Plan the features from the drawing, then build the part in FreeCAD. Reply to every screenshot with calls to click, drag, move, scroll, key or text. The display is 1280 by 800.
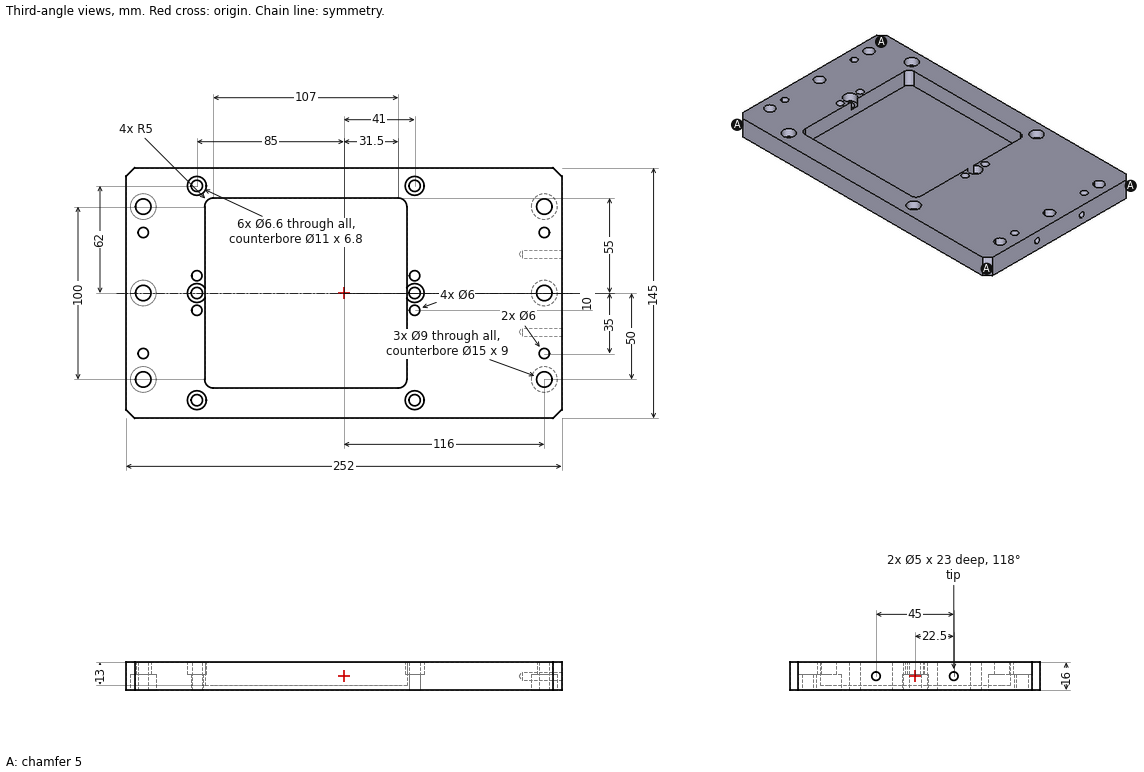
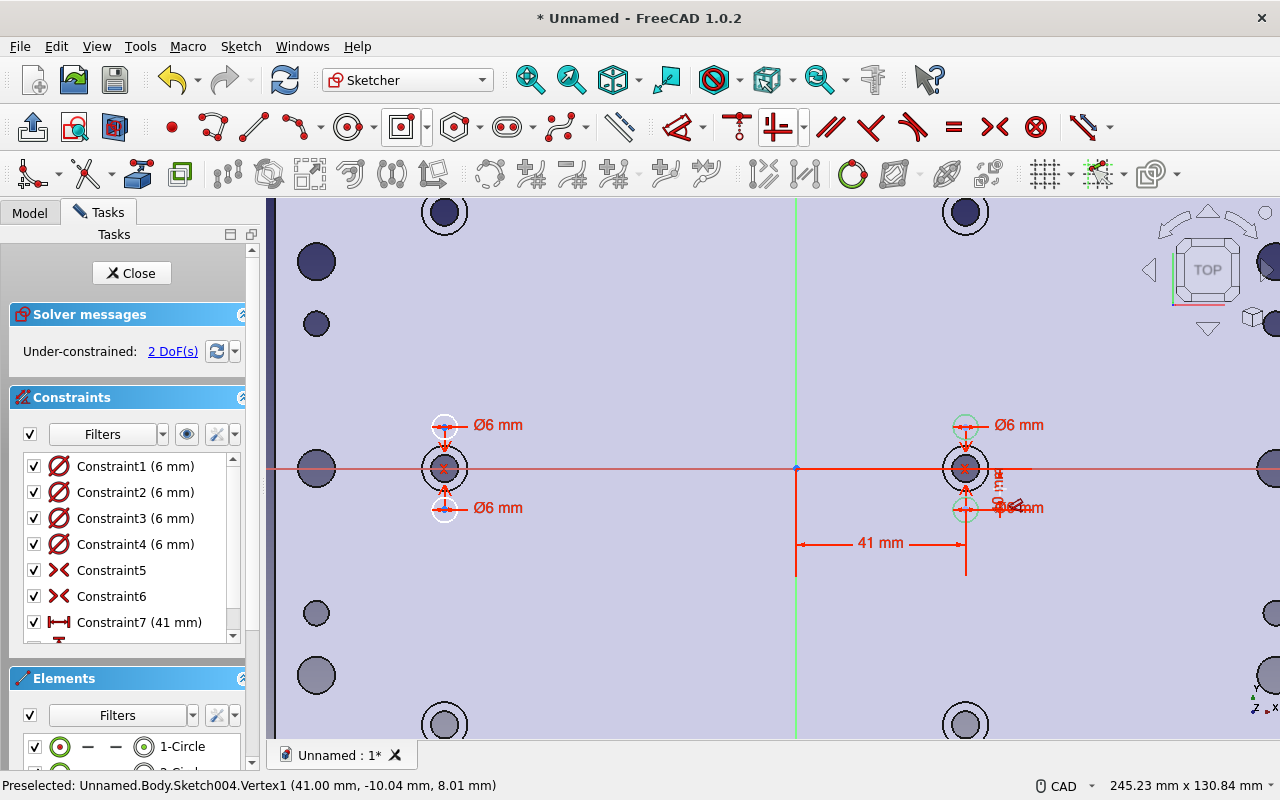
click(445, 510)
click(620, 544)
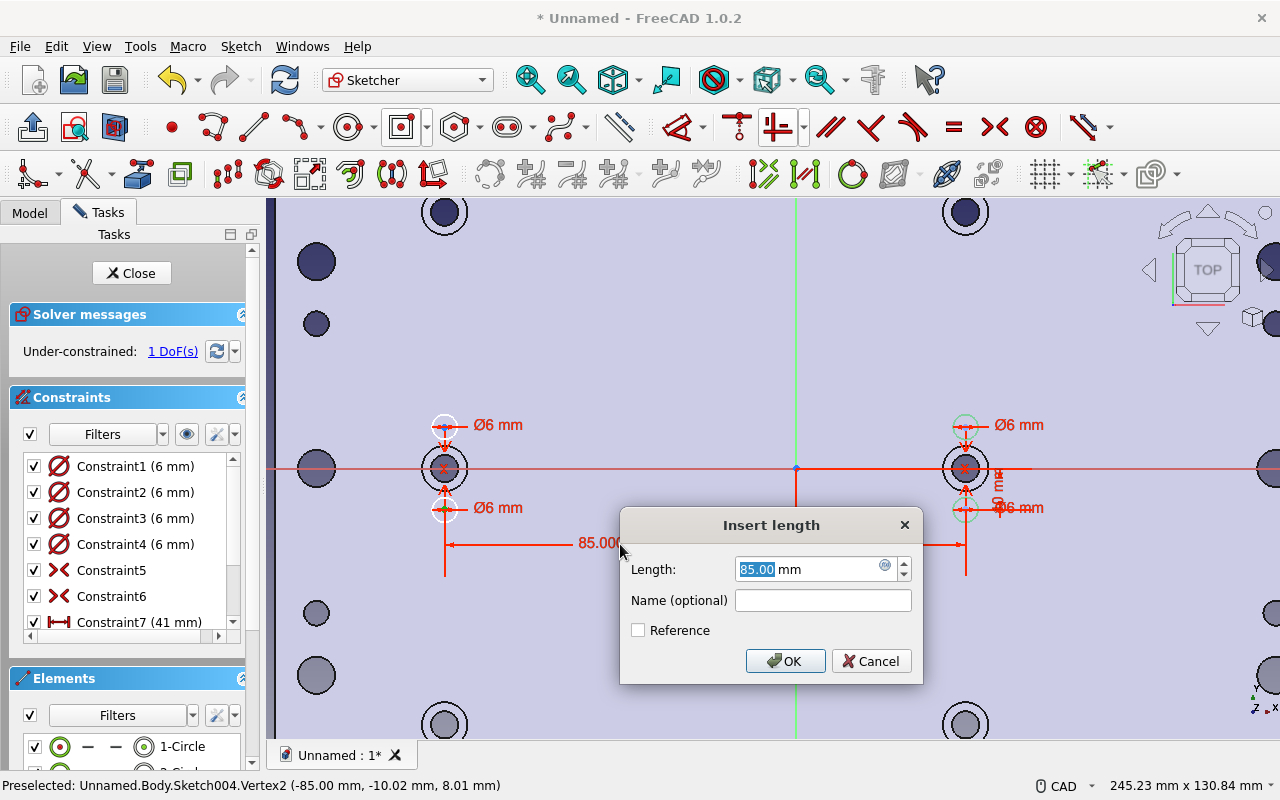
text(85)
key(Return)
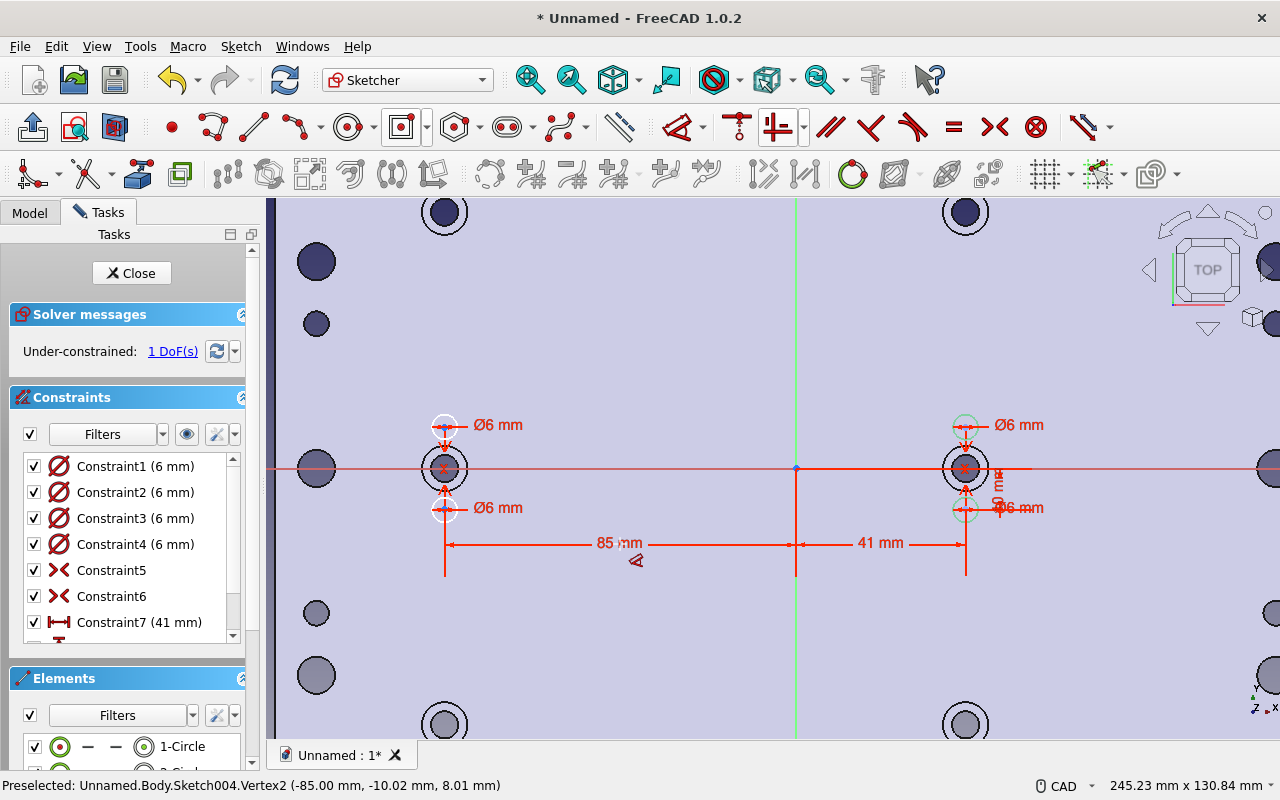
click(445, 510)
click(411, 489)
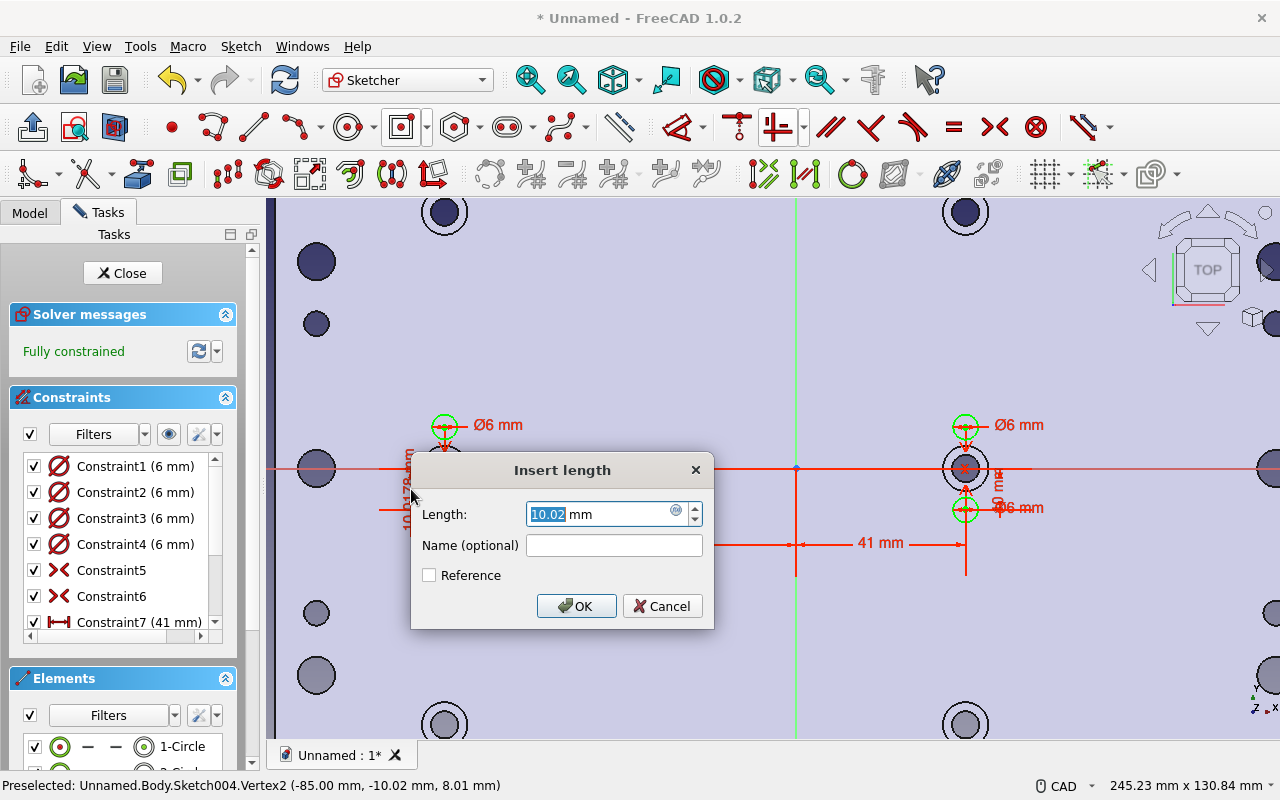
text(10)
key(Return)
key(Escape)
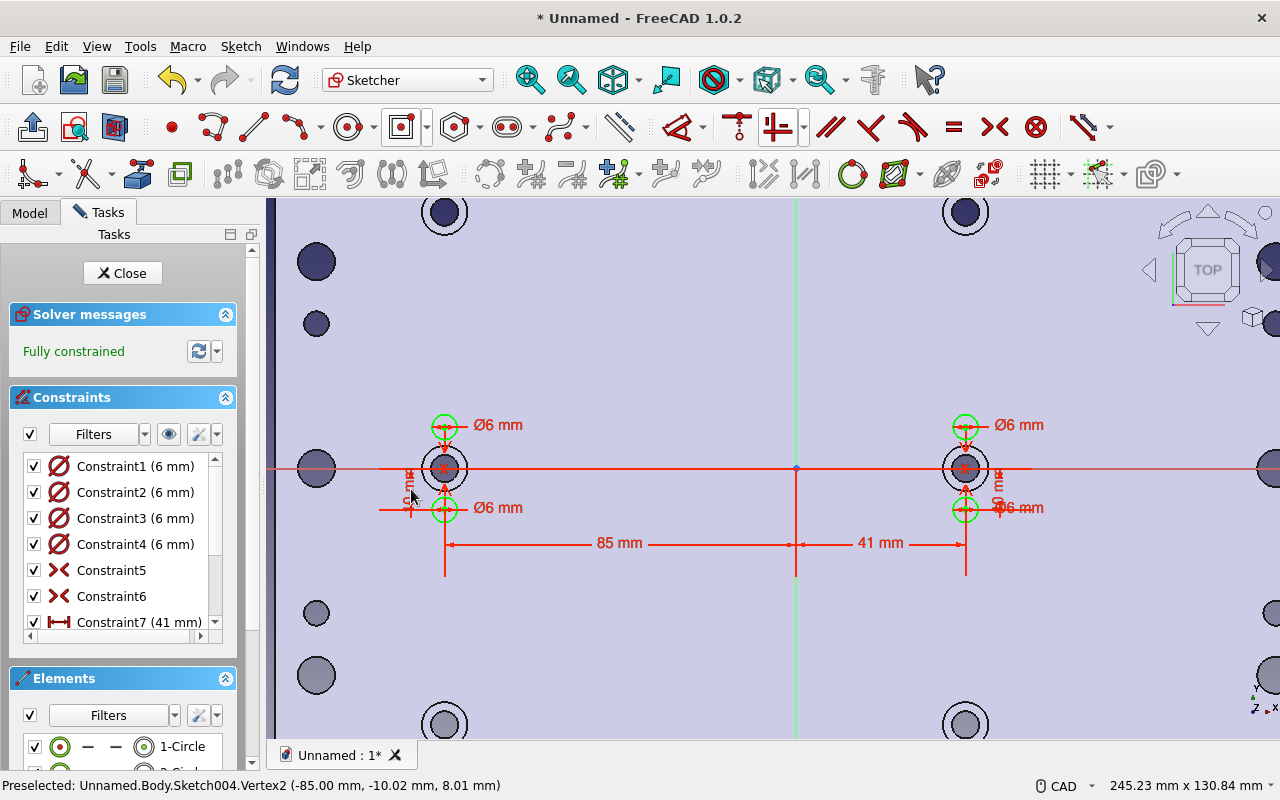
click(123, 273)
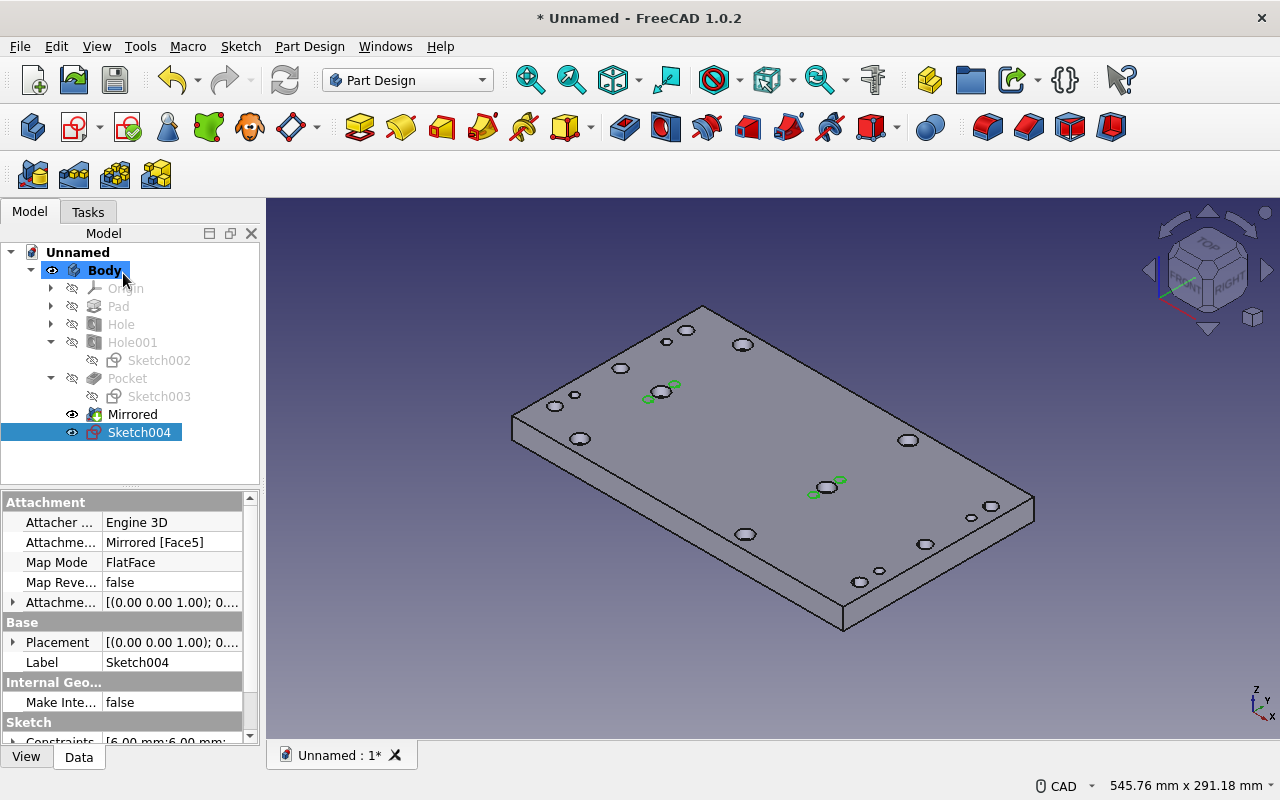
click(625, 128)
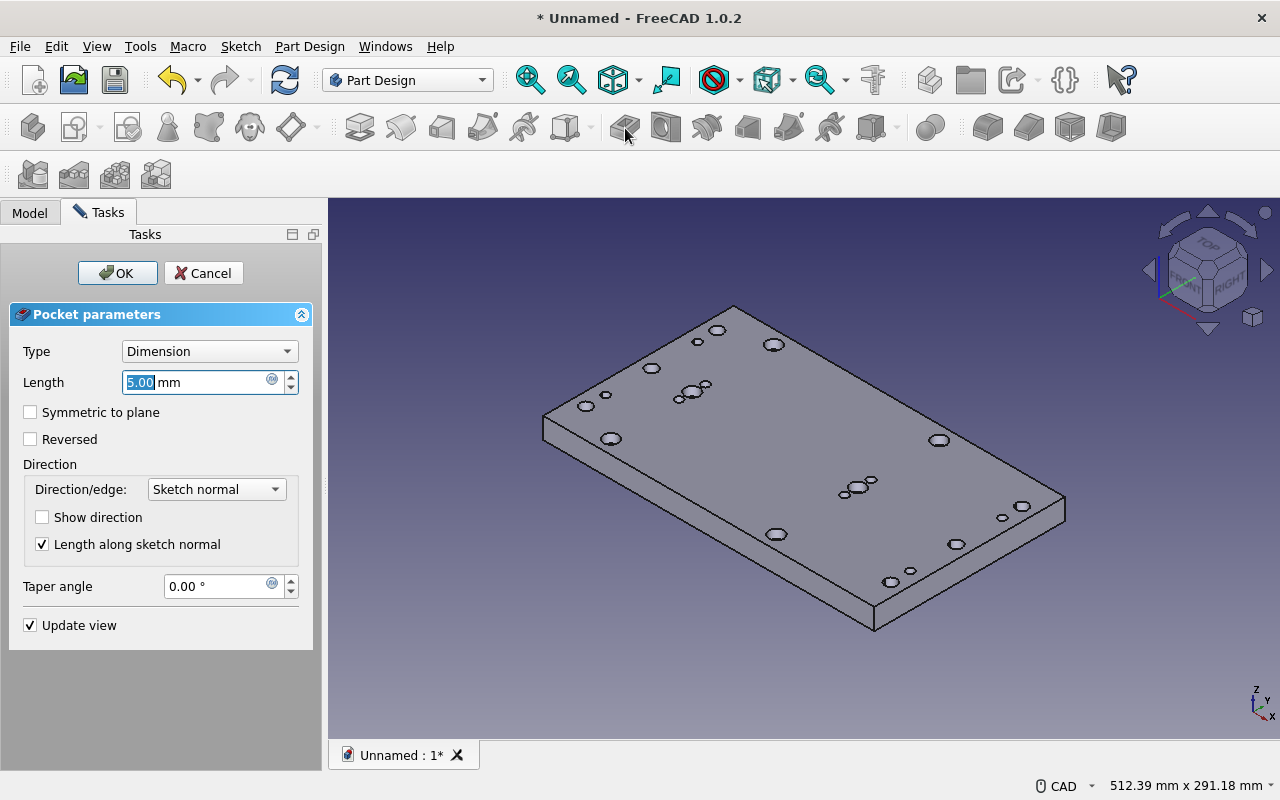
click(210, 352)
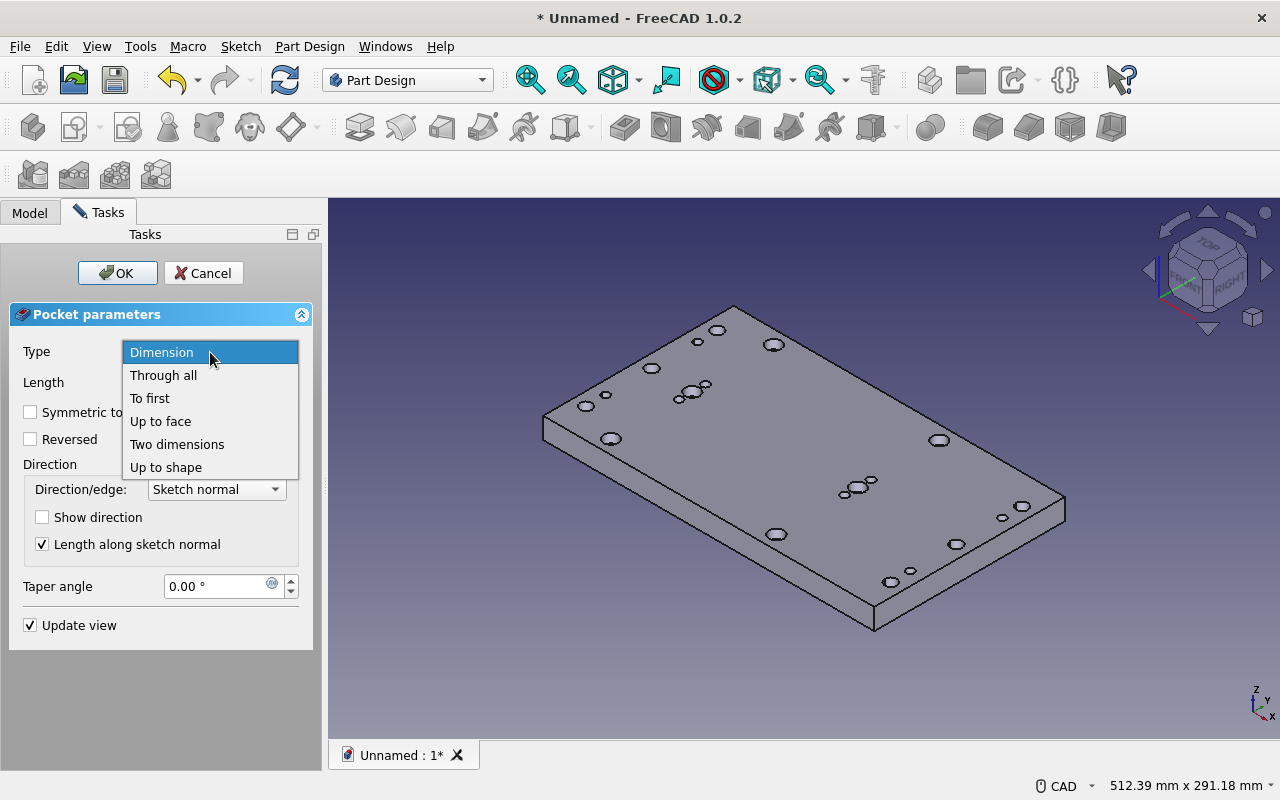
click(208, 376)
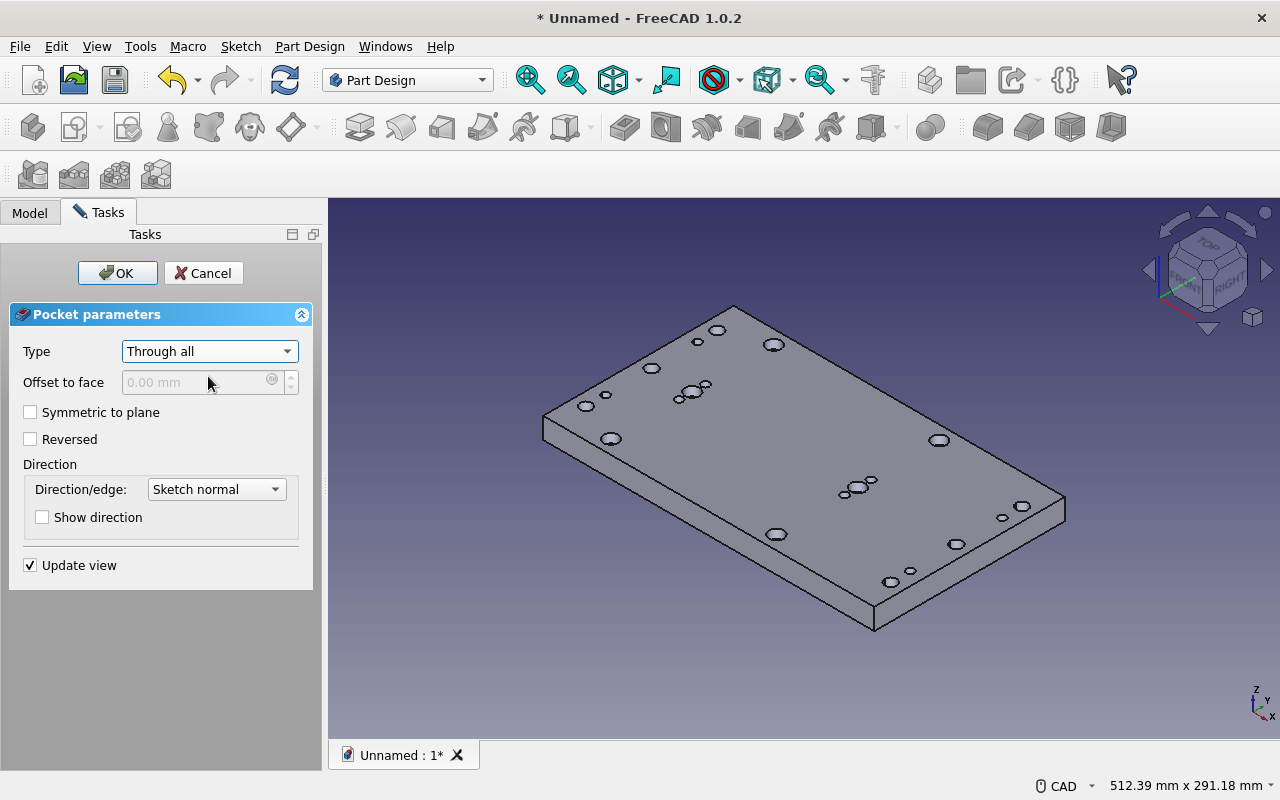
click(118, 273)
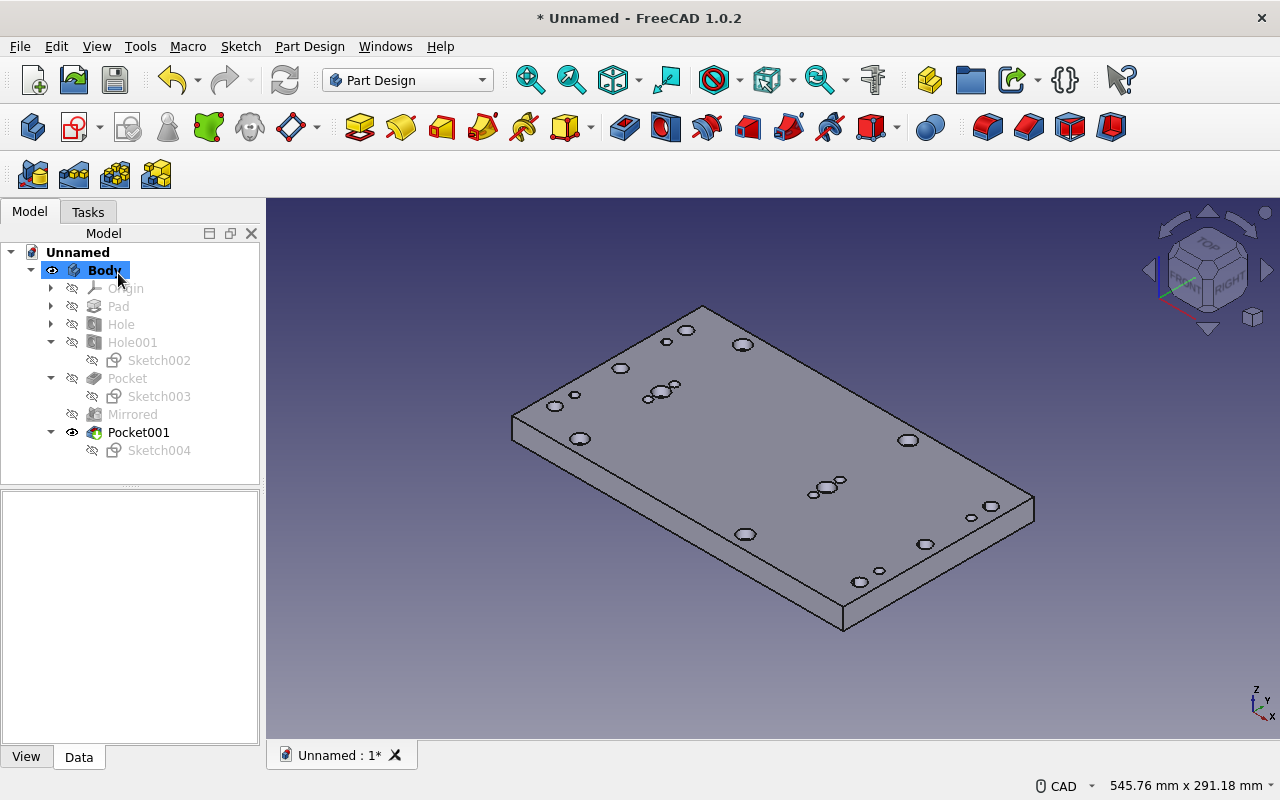
click(698, 444)